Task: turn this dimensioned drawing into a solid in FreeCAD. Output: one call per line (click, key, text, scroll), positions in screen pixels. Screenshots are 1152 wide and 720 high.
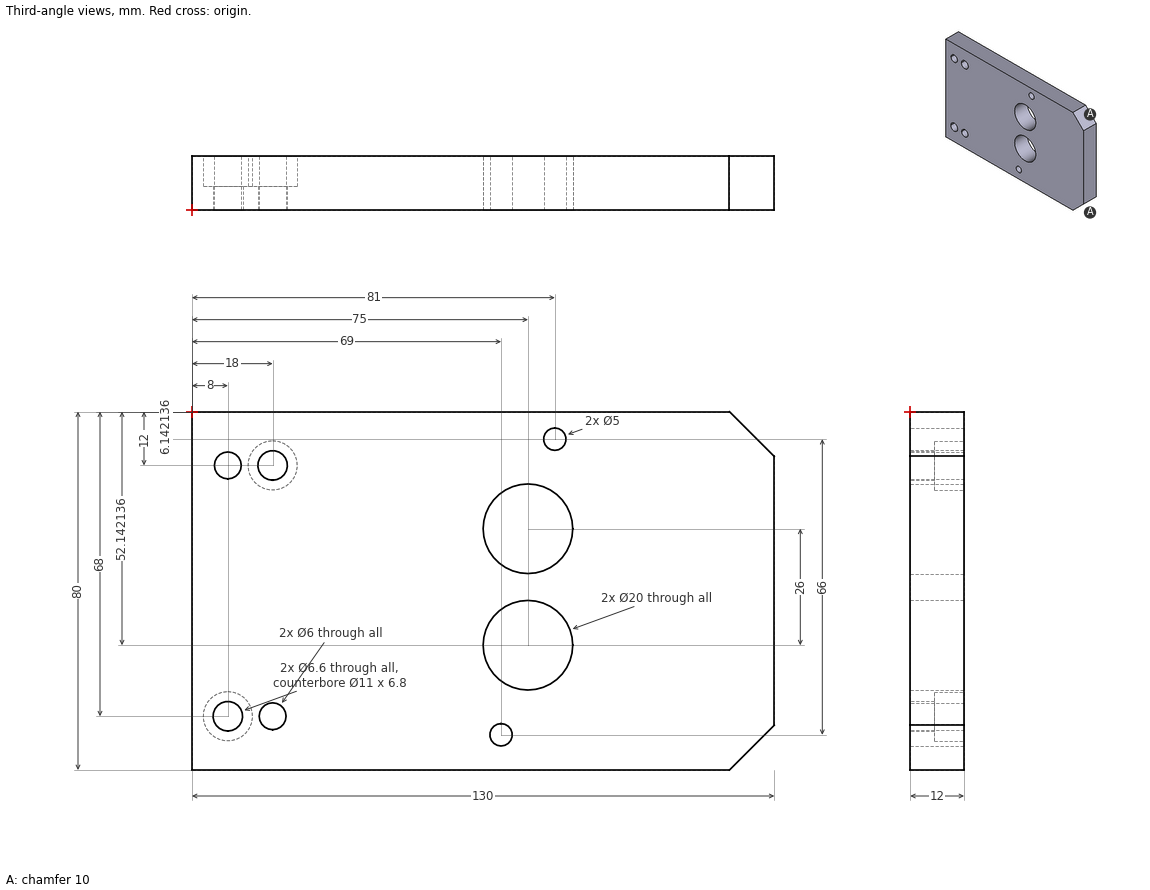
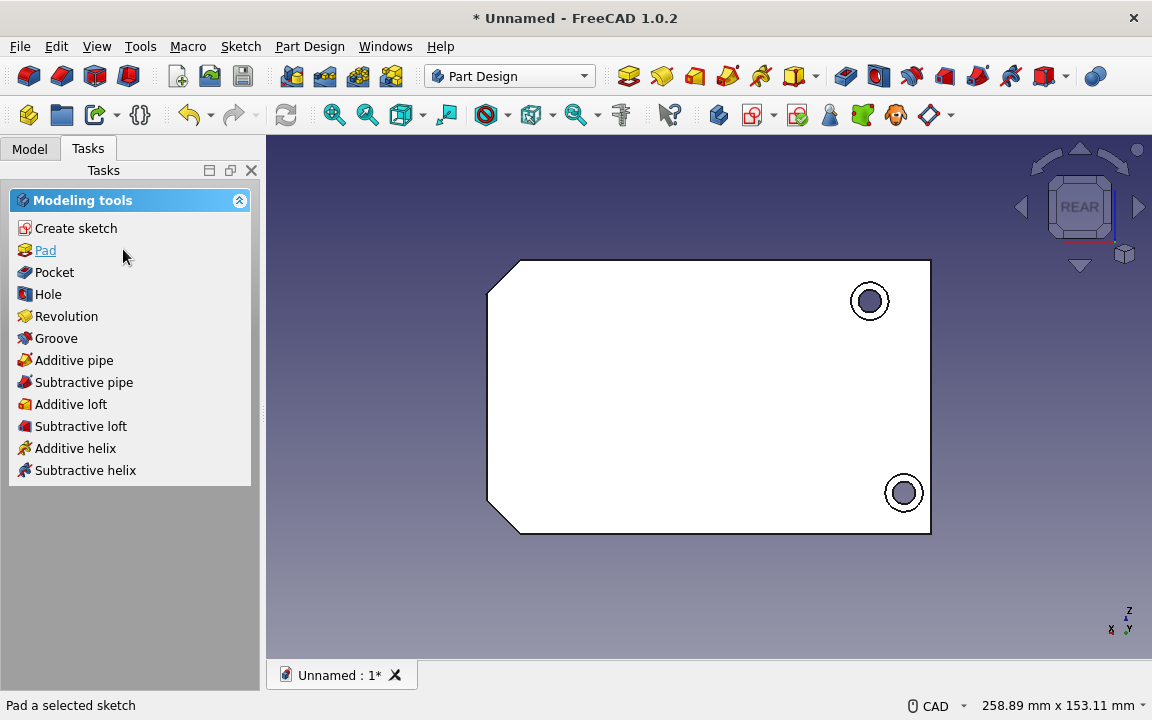
click(879, 76)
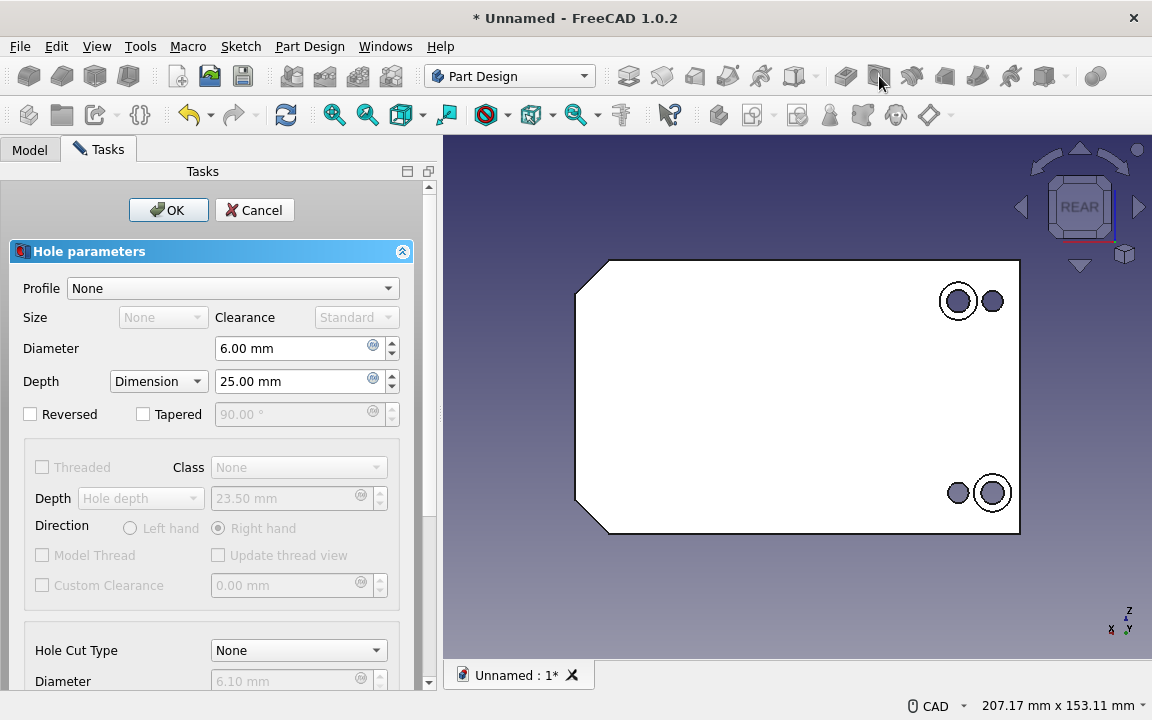
triple_click(300, 348)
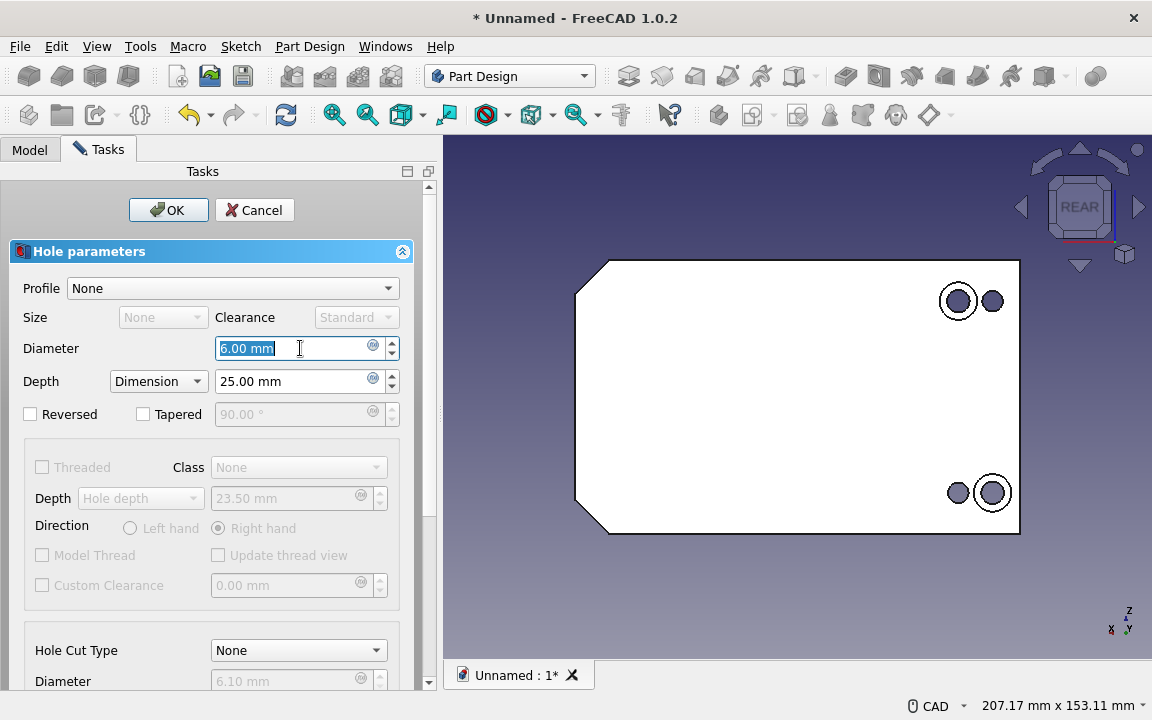
text(6)
key(Tab)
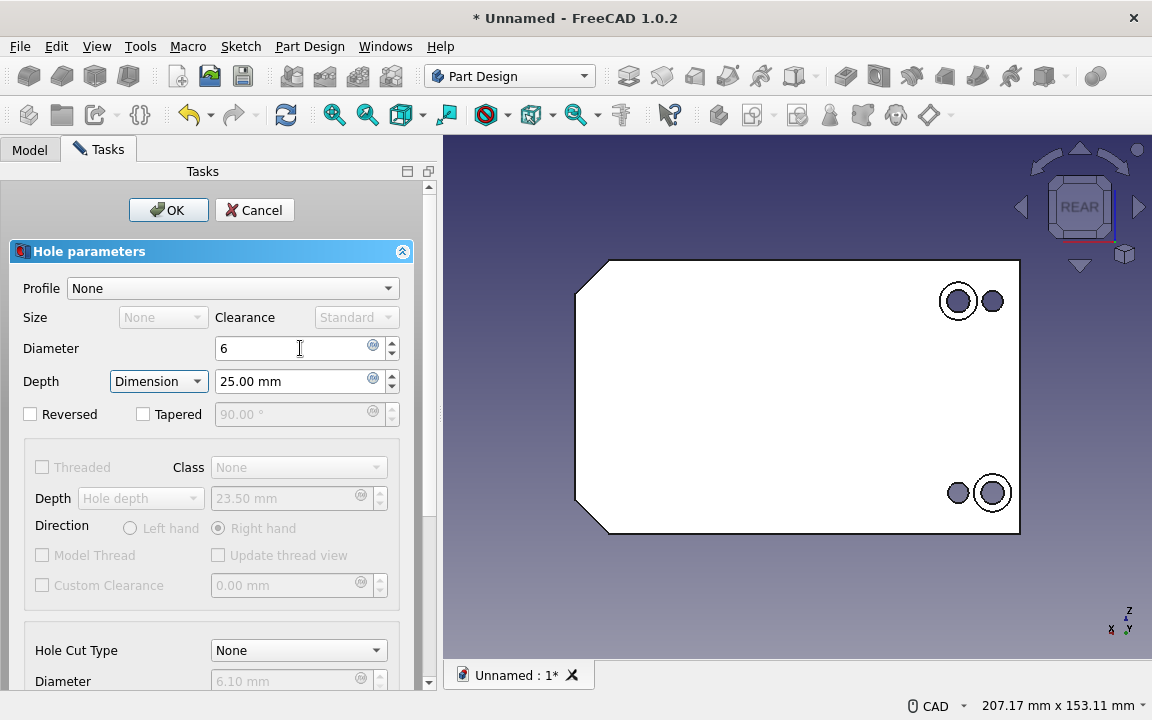
click(160, 382)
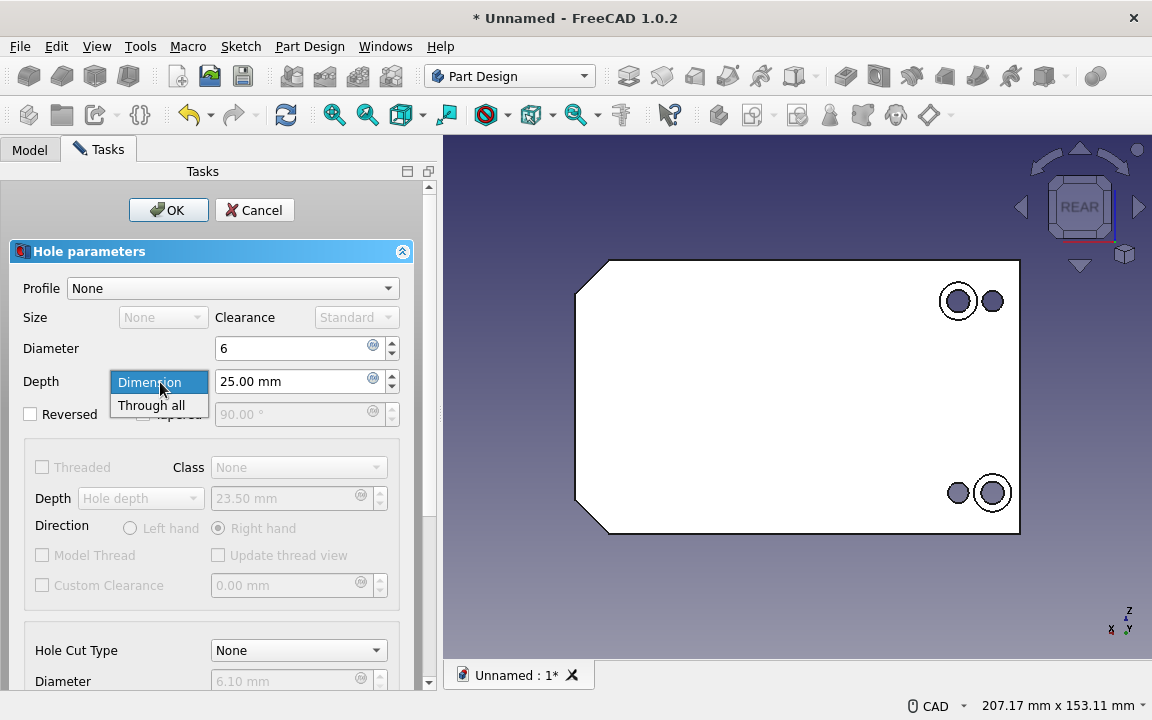
click(158, 406)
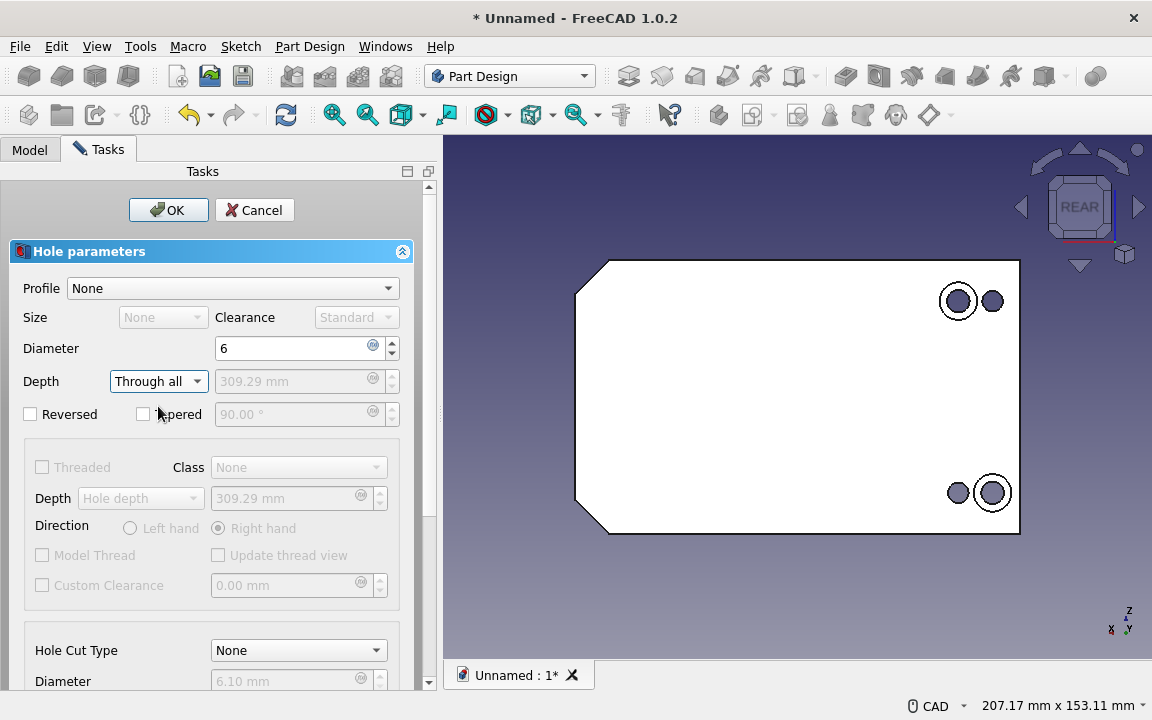
click(169, 210)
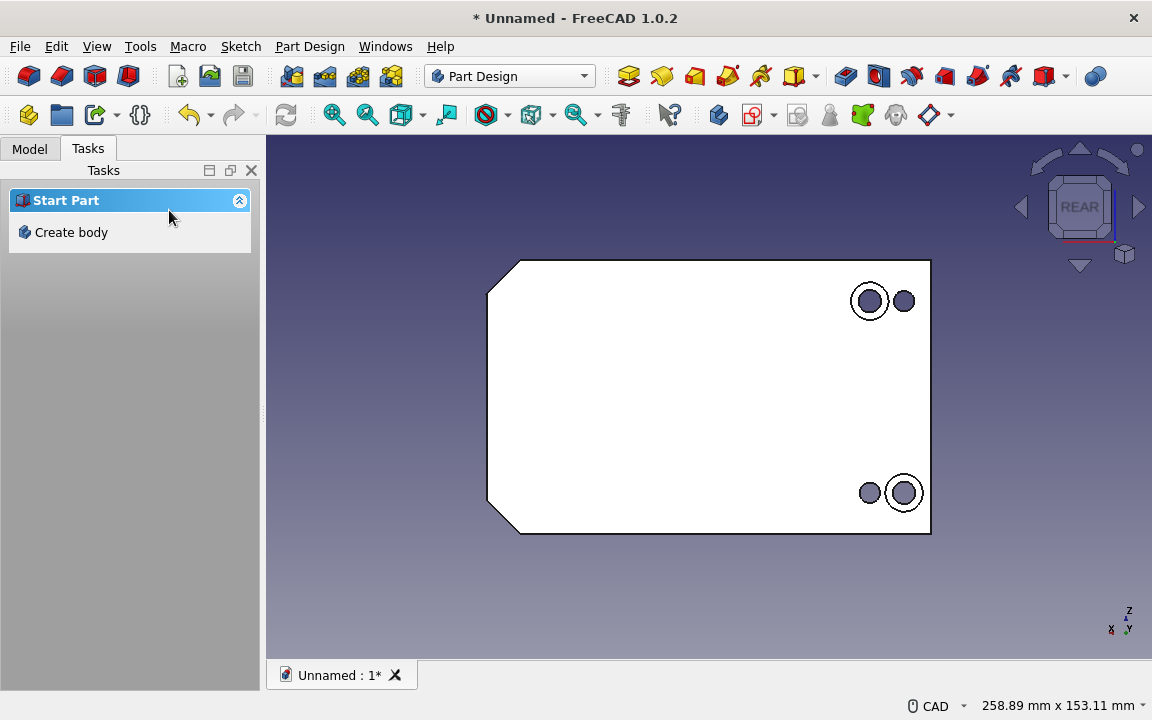
click(752, 116)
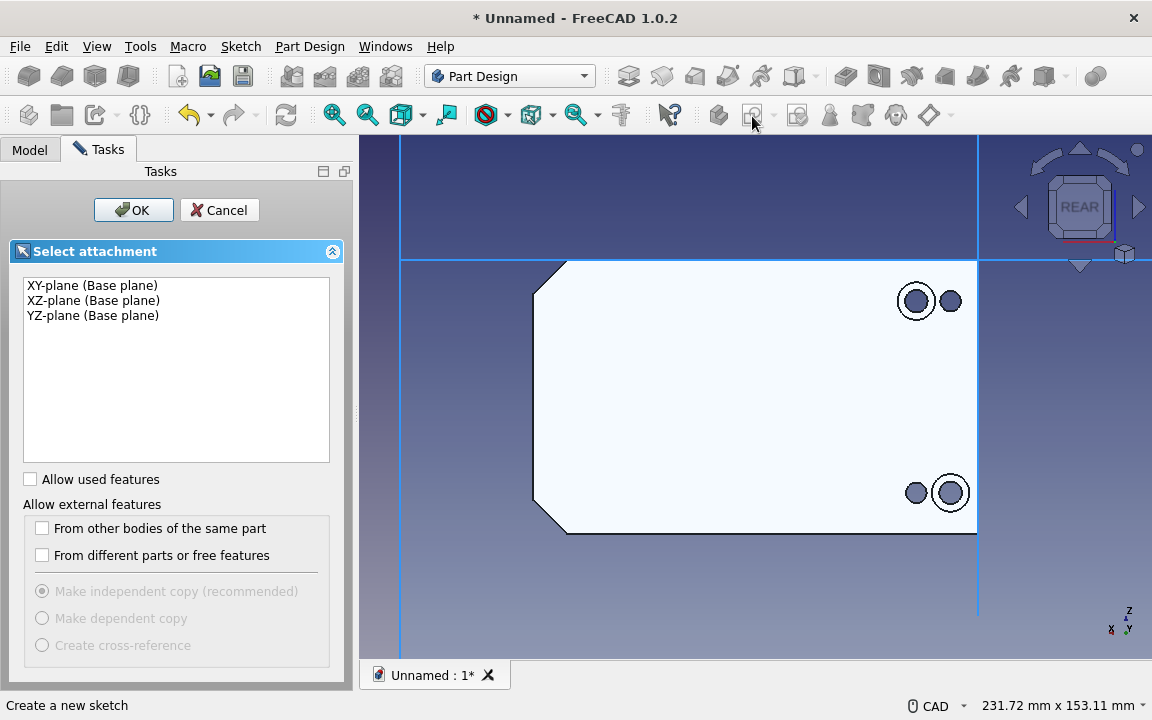
click(84, 300)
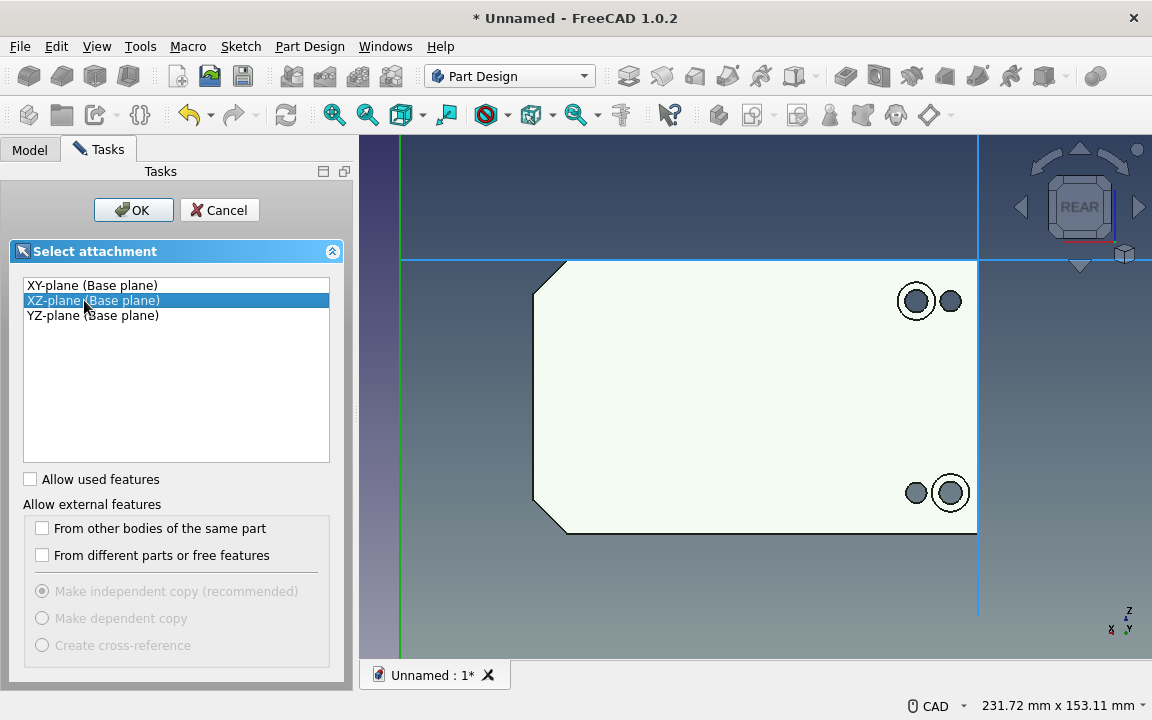
click(134, 210)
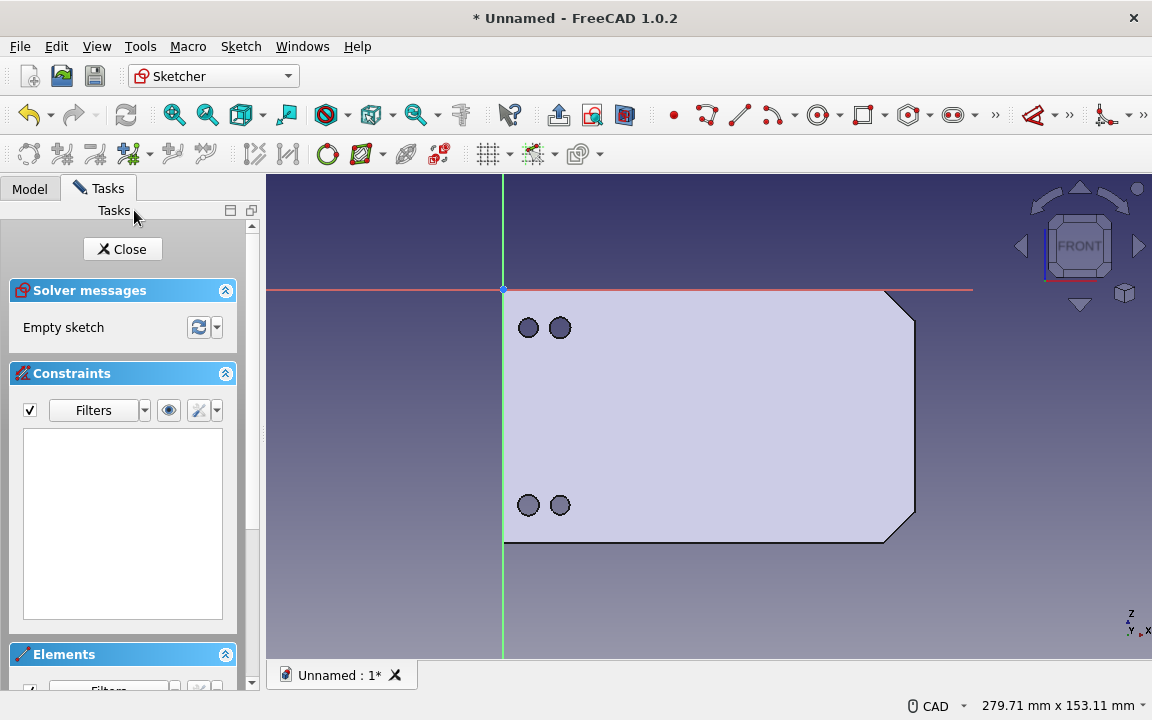
scroll(632, 331, up, 2)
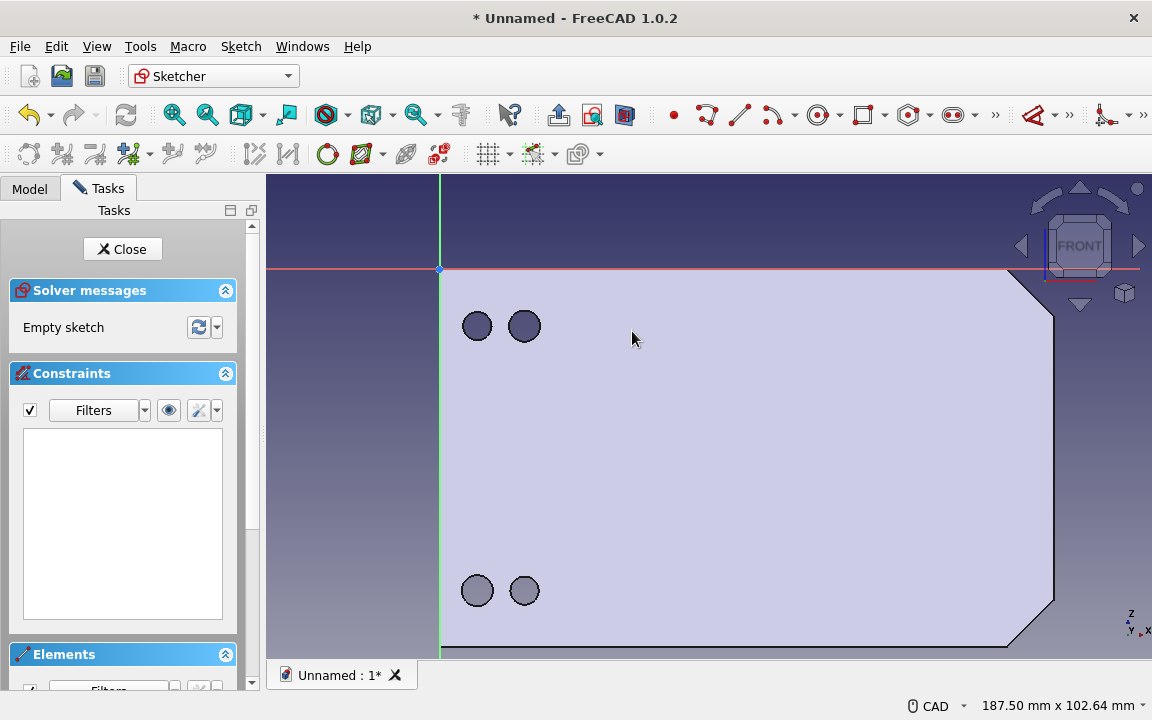
key(g)
key(c)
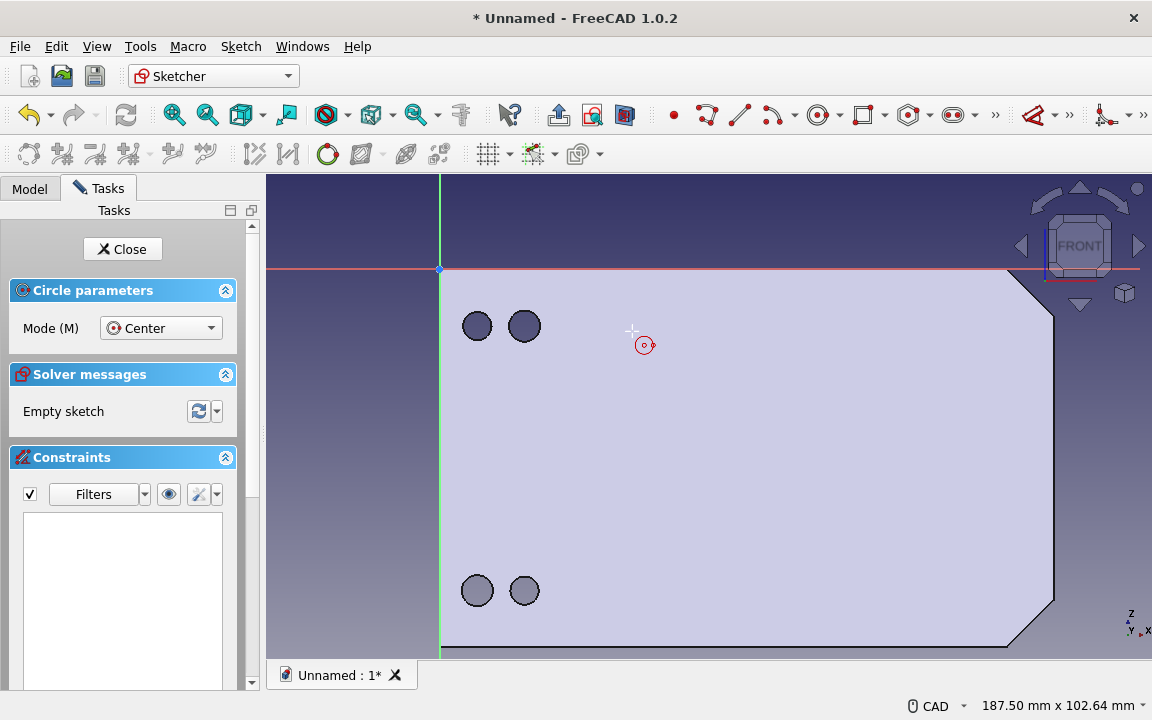
click(794, 516)
click(827, 482)